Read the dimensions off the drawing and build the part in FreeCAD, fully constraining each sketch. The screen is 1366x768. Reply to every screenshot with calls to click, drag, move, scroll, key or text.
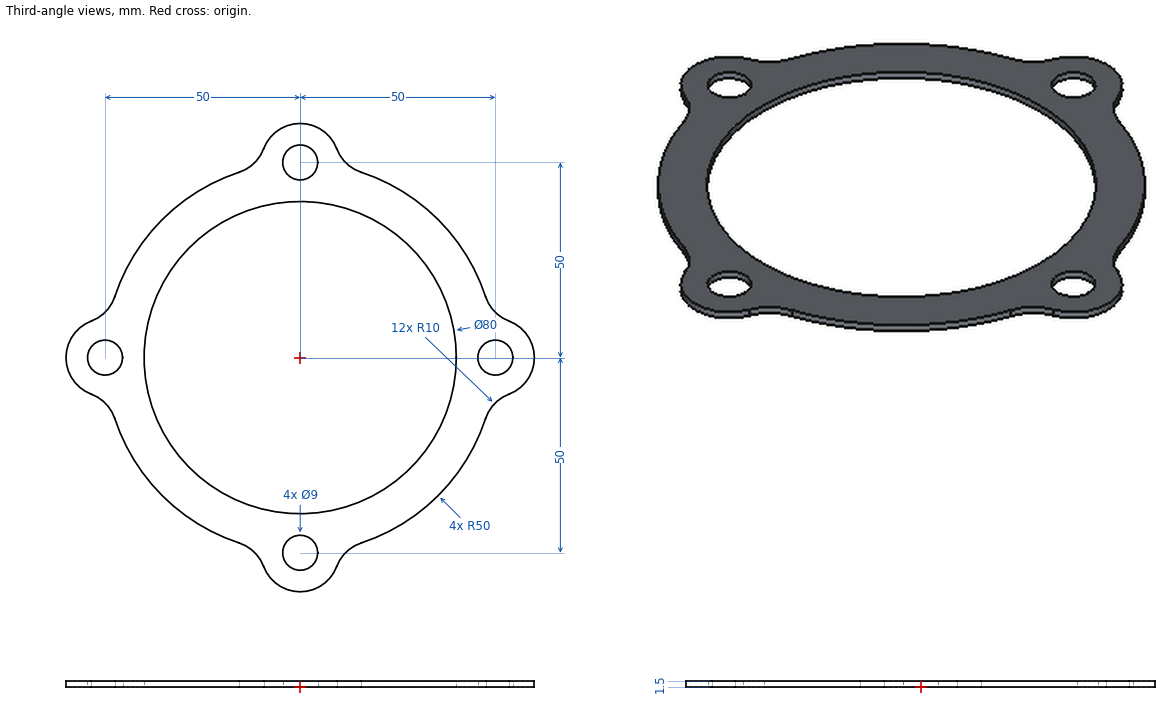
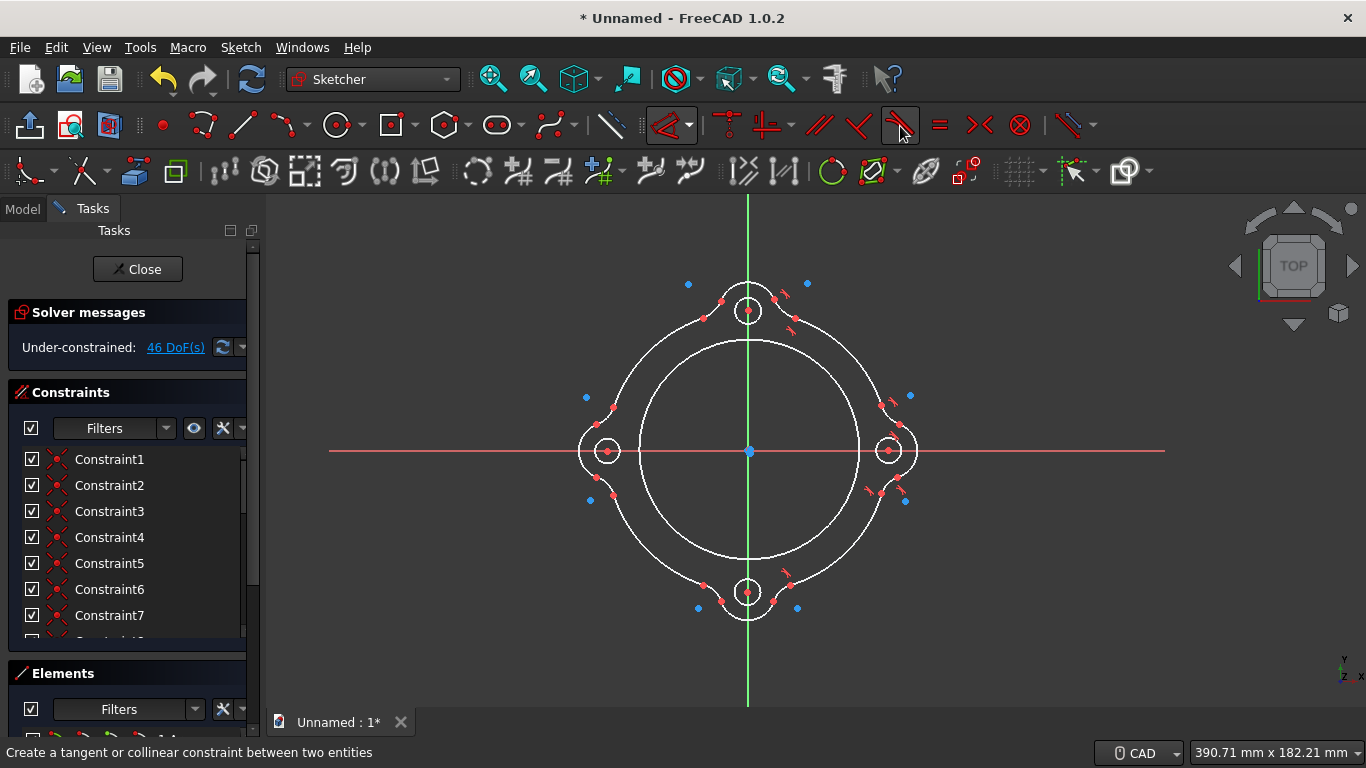
click(760, 285)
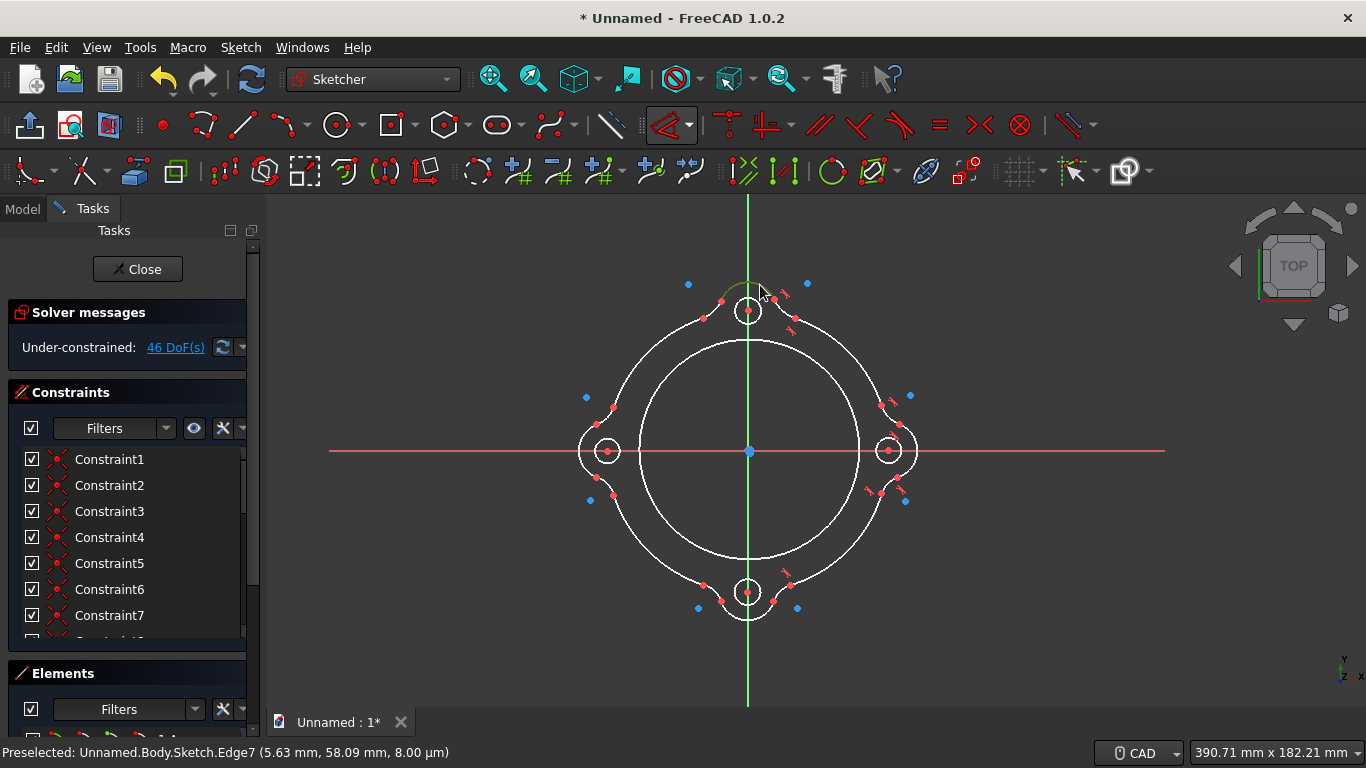
click(714, 311)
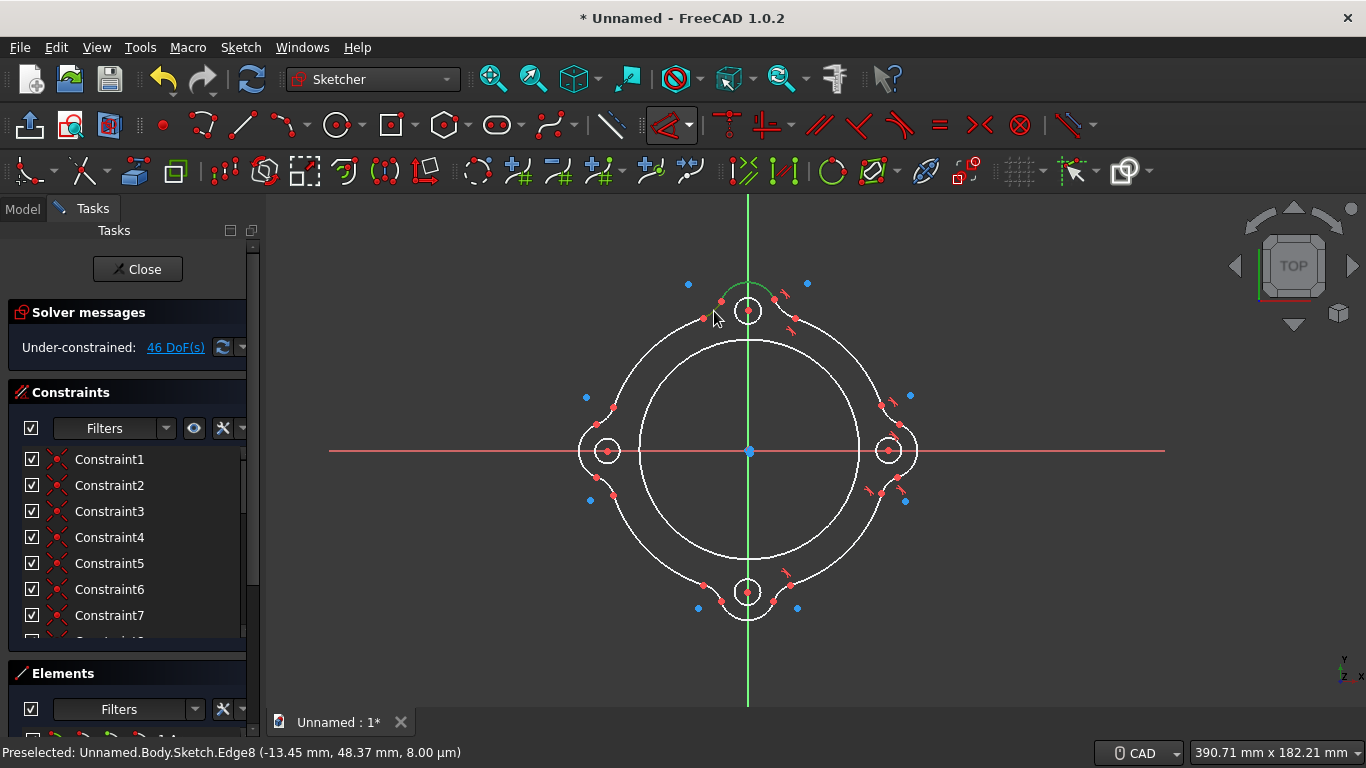
click(900, 126)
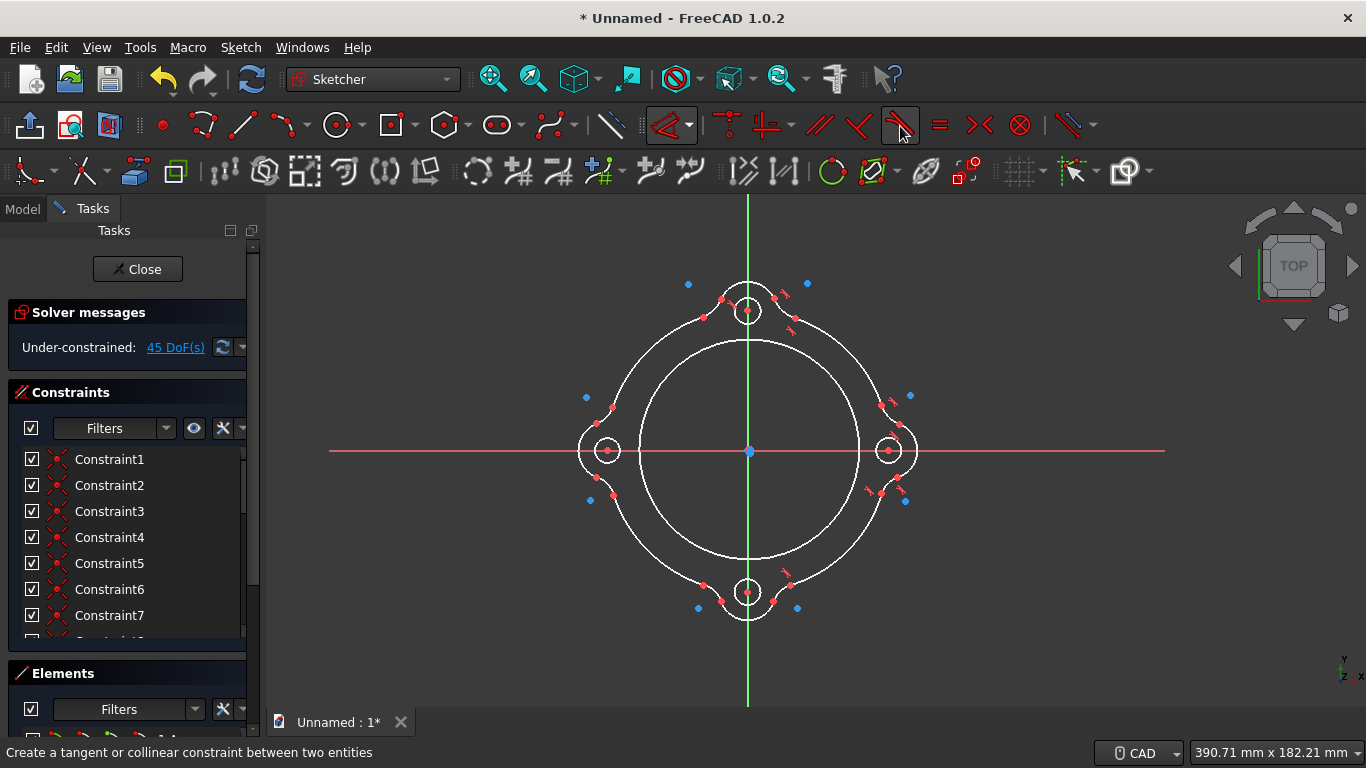
click(714, 310)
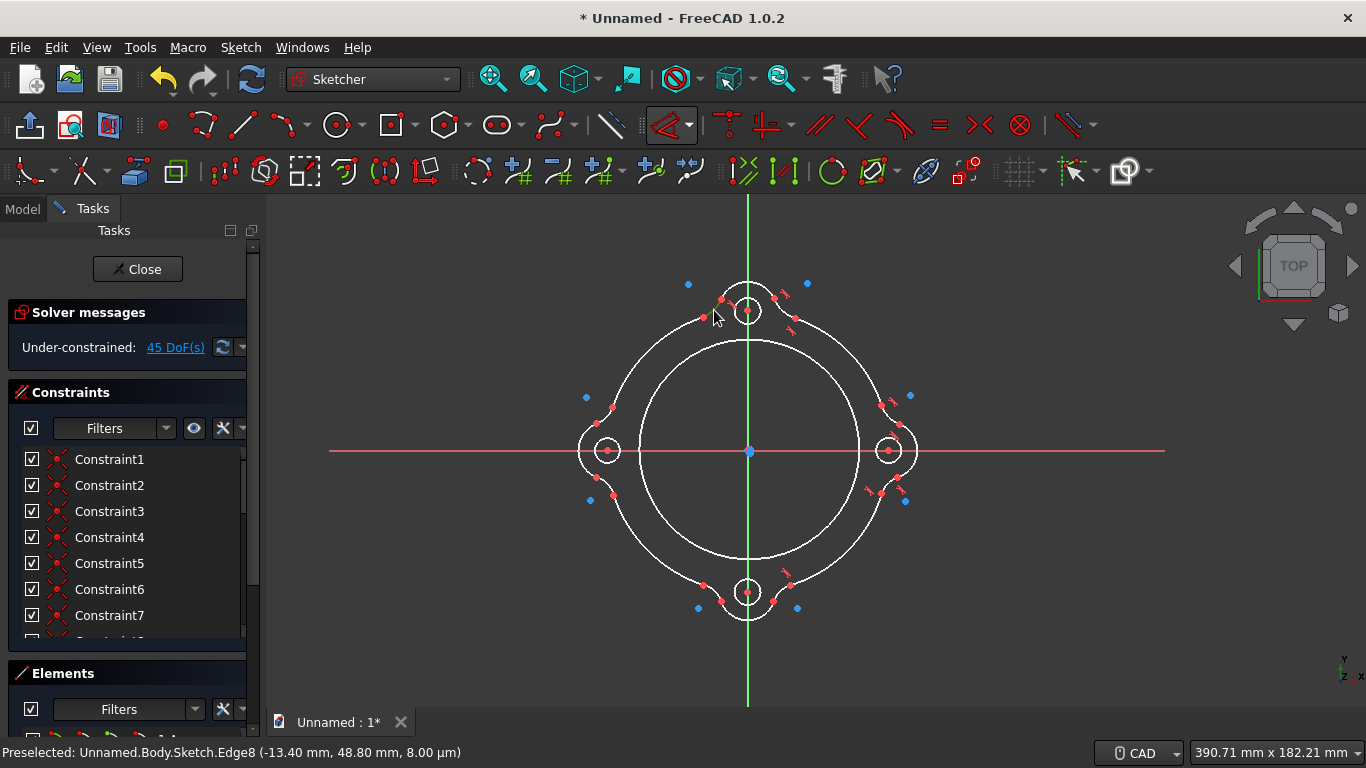
click(668, 335)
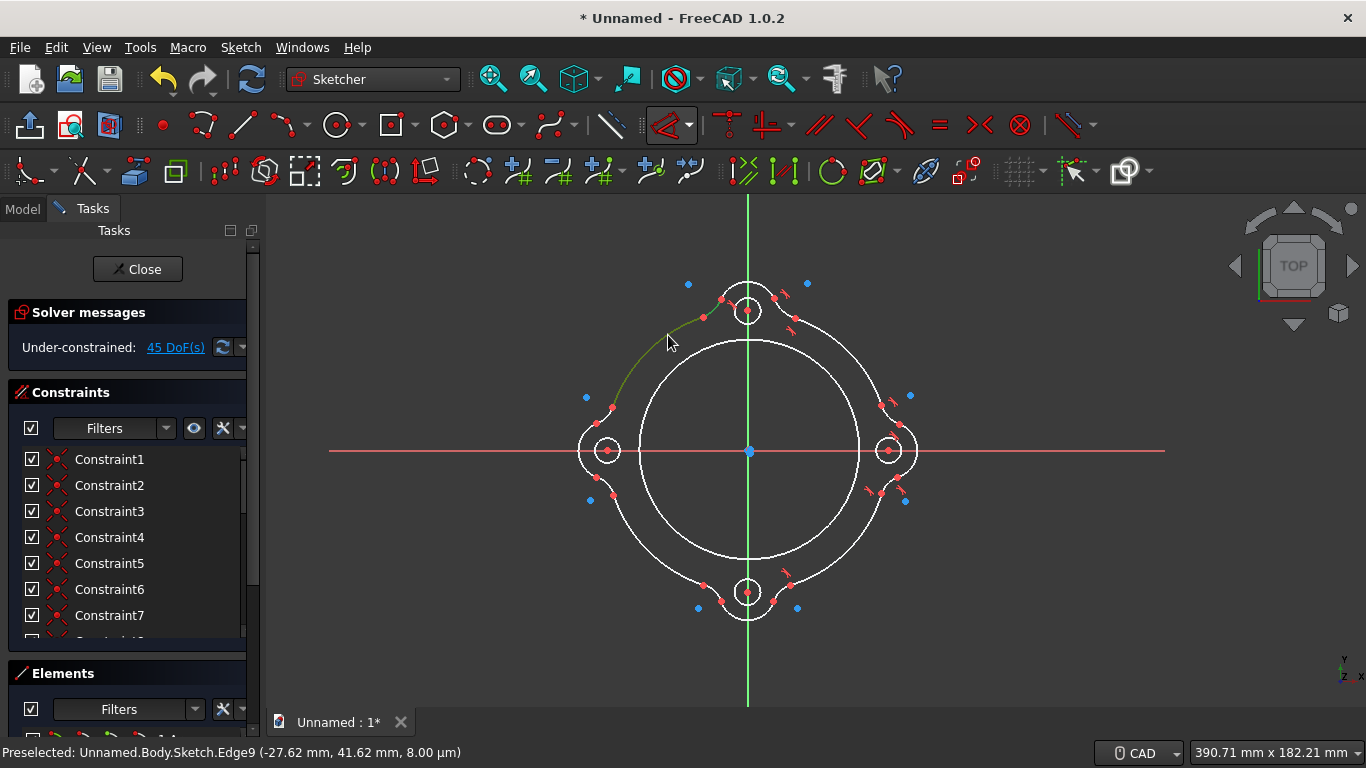
click(900, 126)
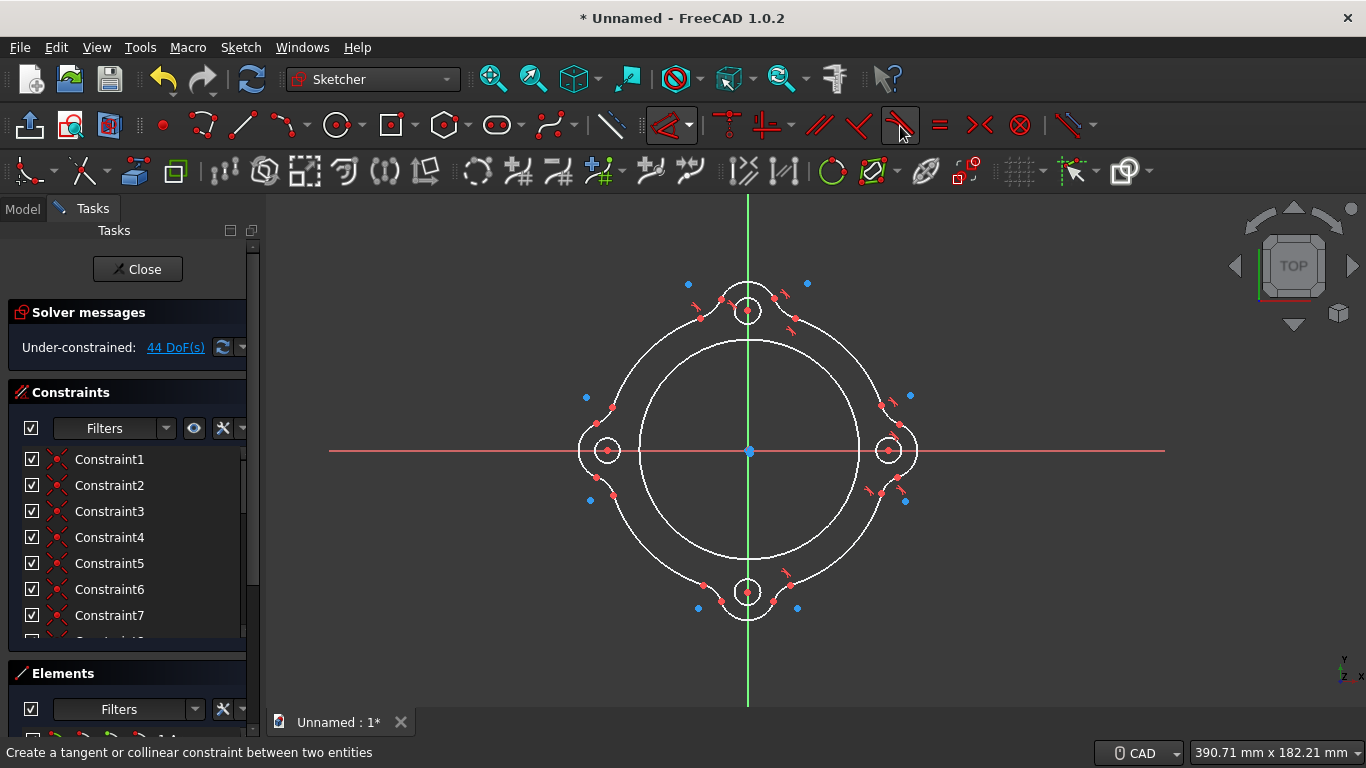
click(666, 336)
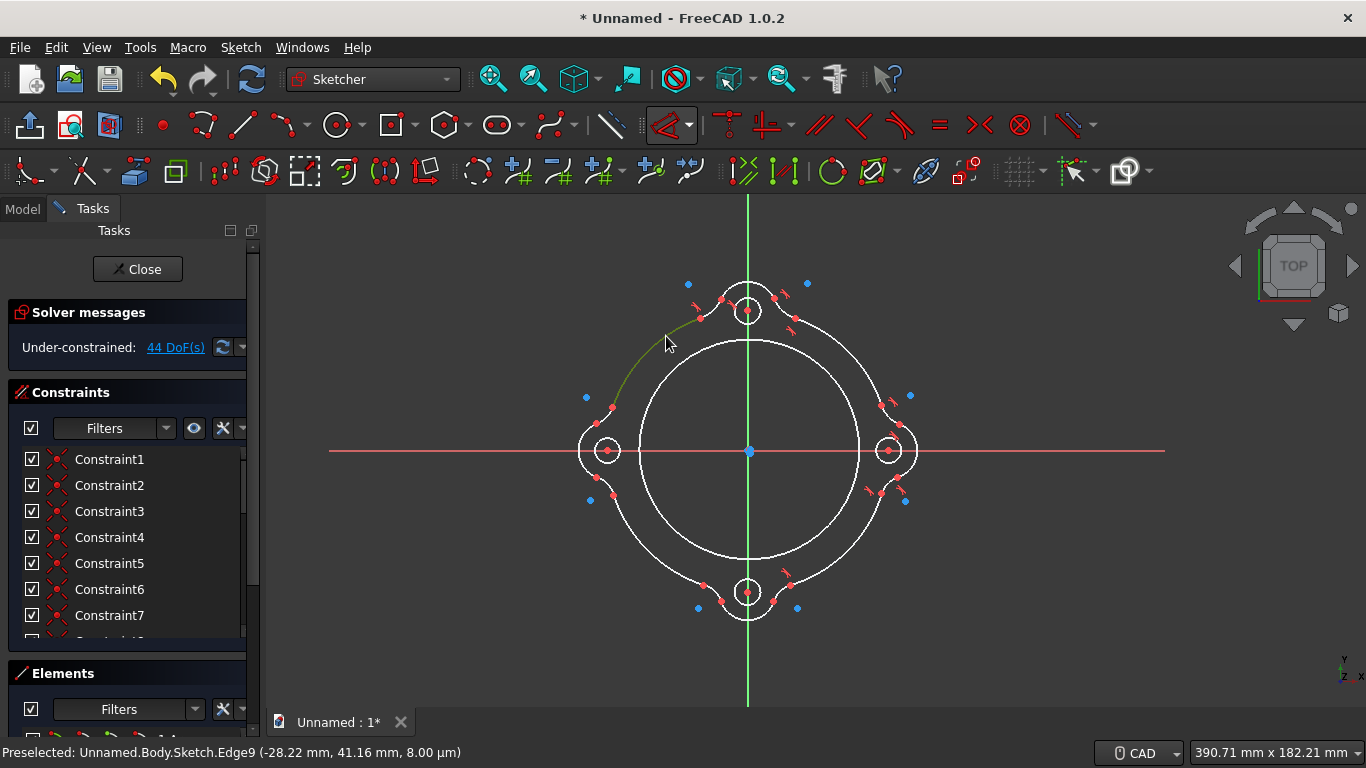
click(606, 417)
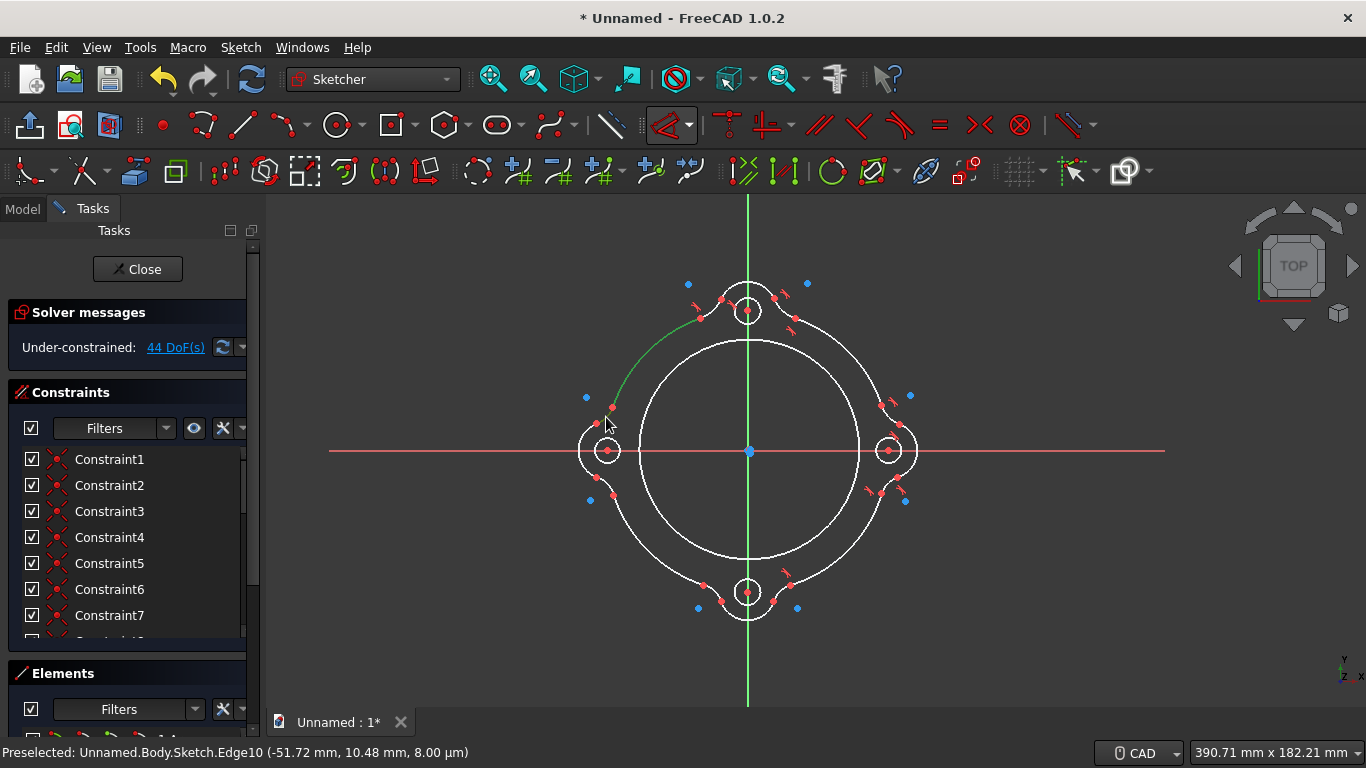
click(900, 126)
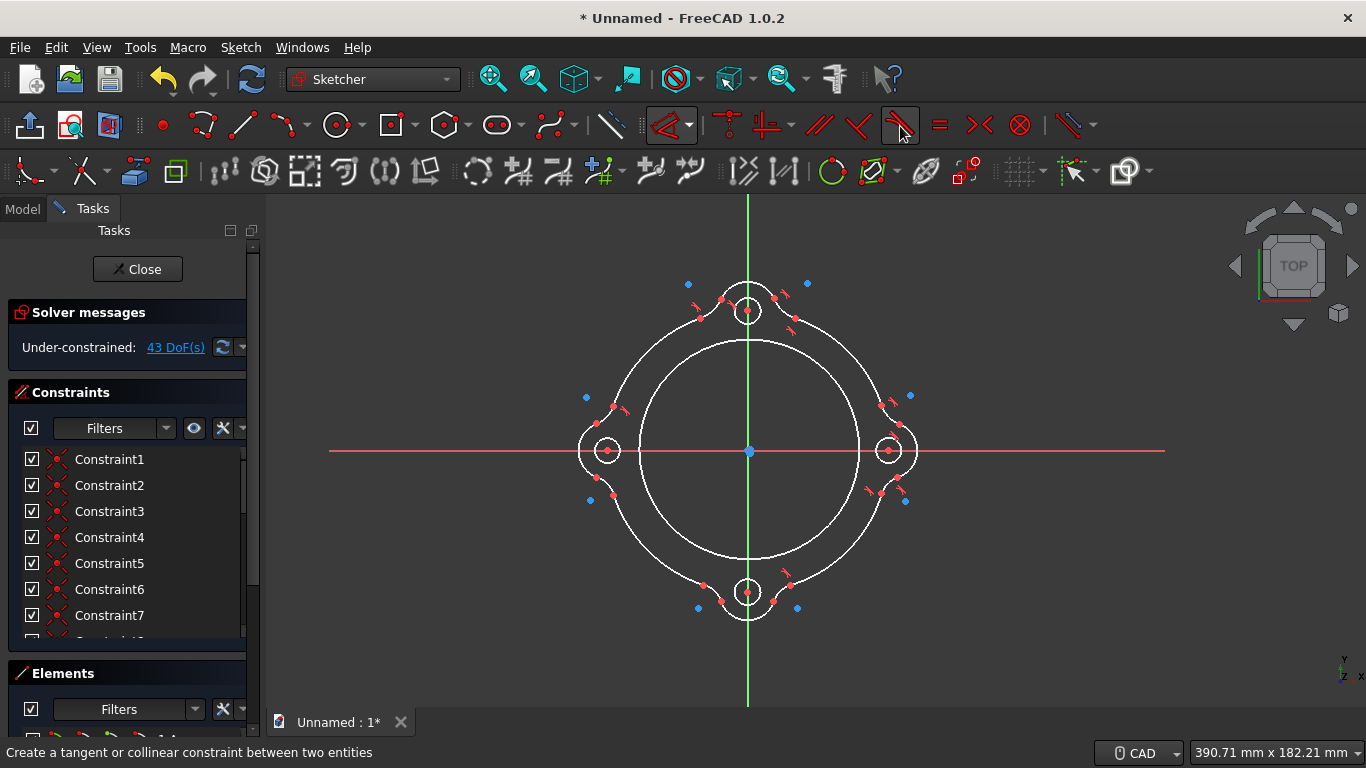
click(607, 417)